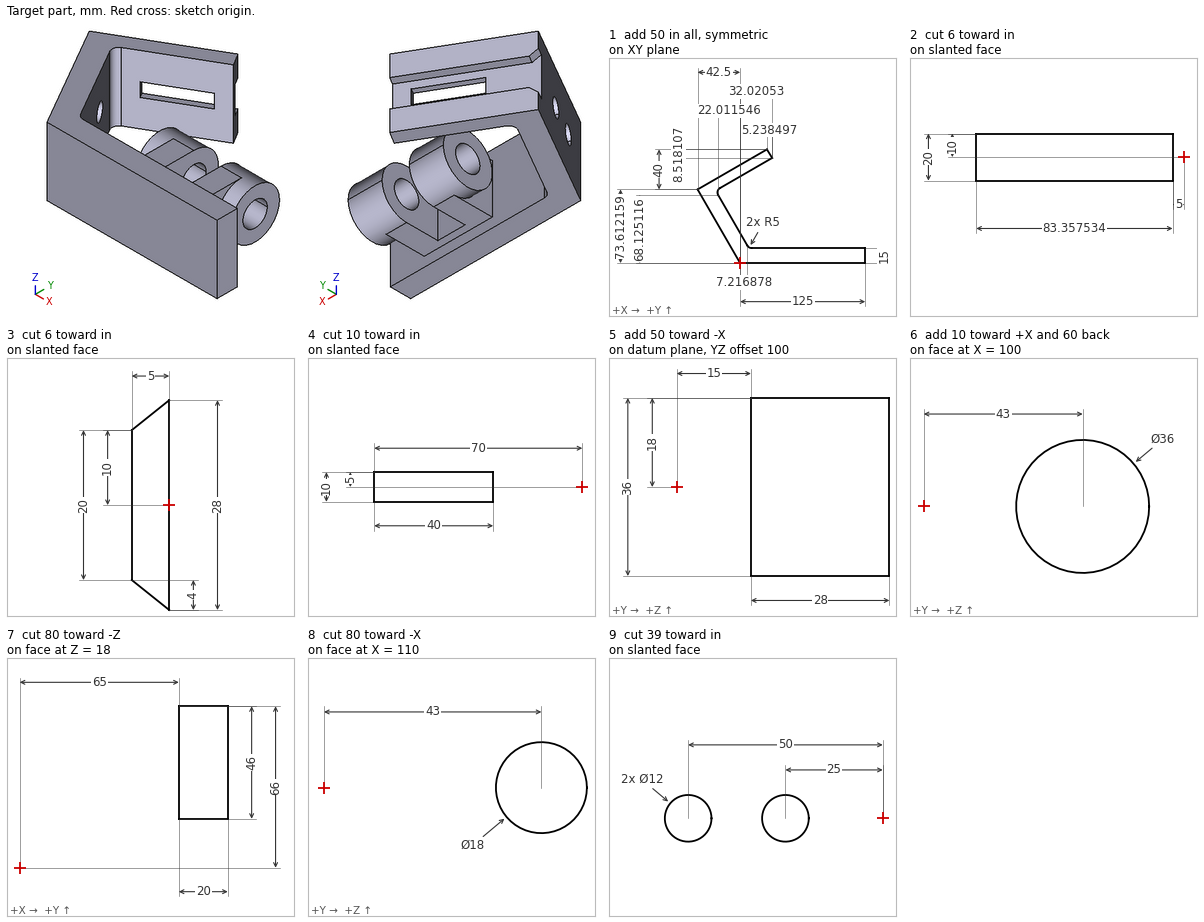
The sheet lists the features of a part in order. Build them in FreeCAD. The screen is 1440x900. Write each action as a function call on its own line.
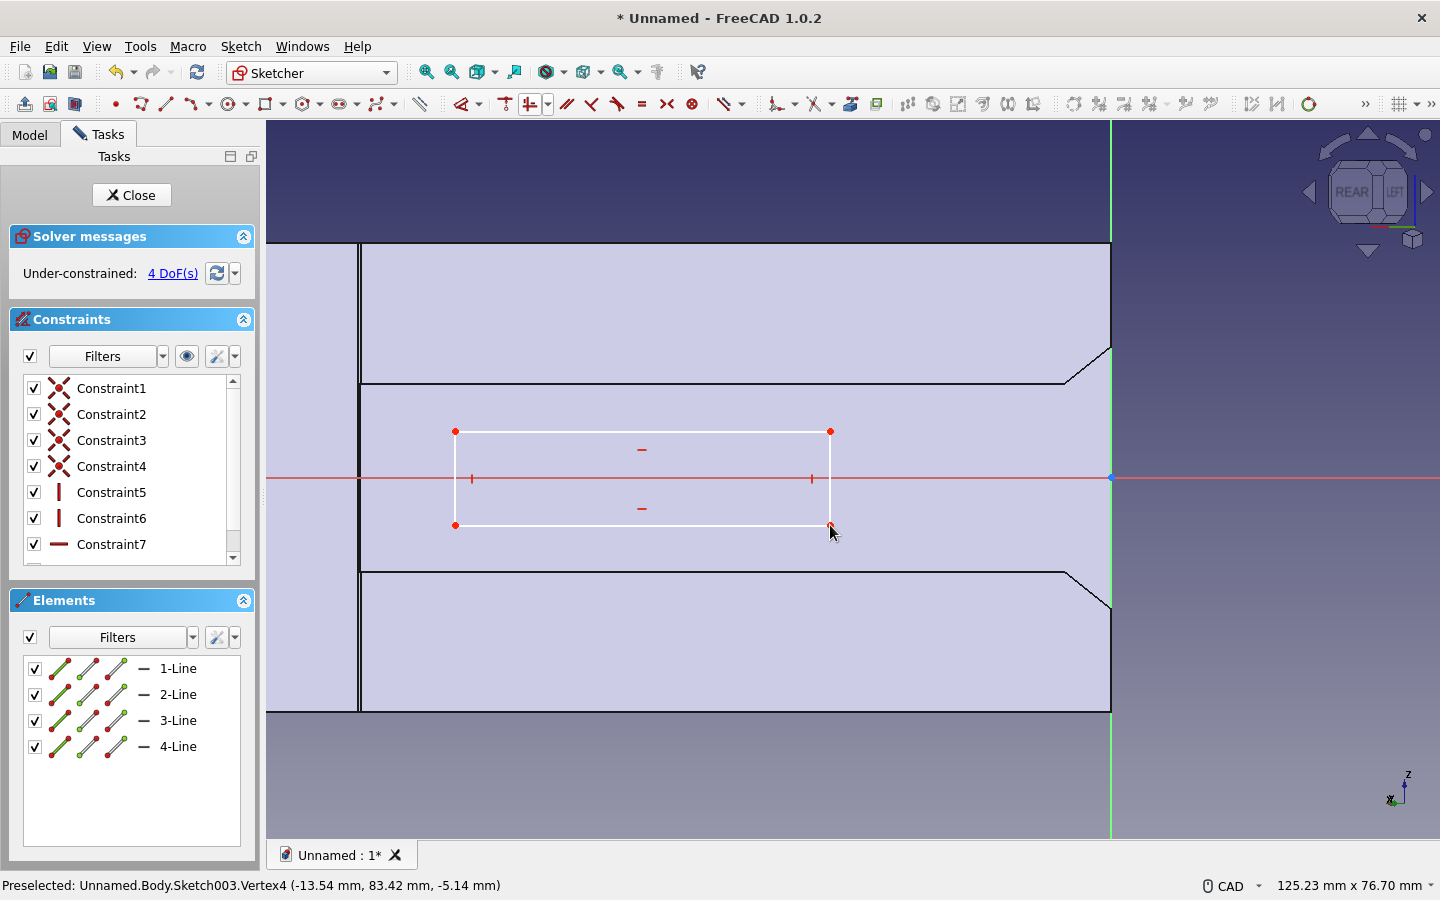
key(d)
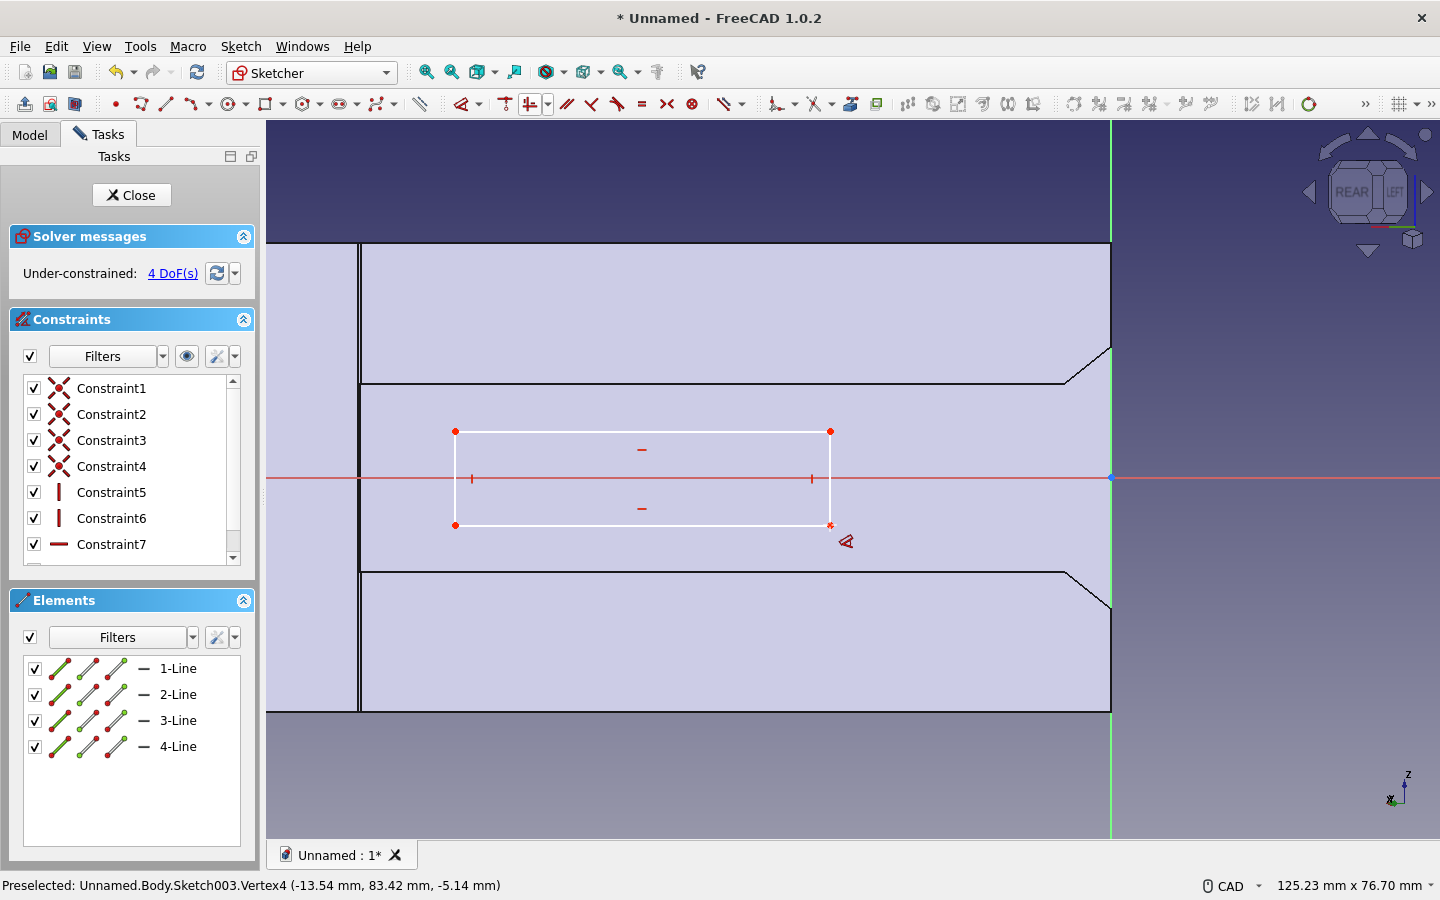
click(455, 460)
click(421, 457)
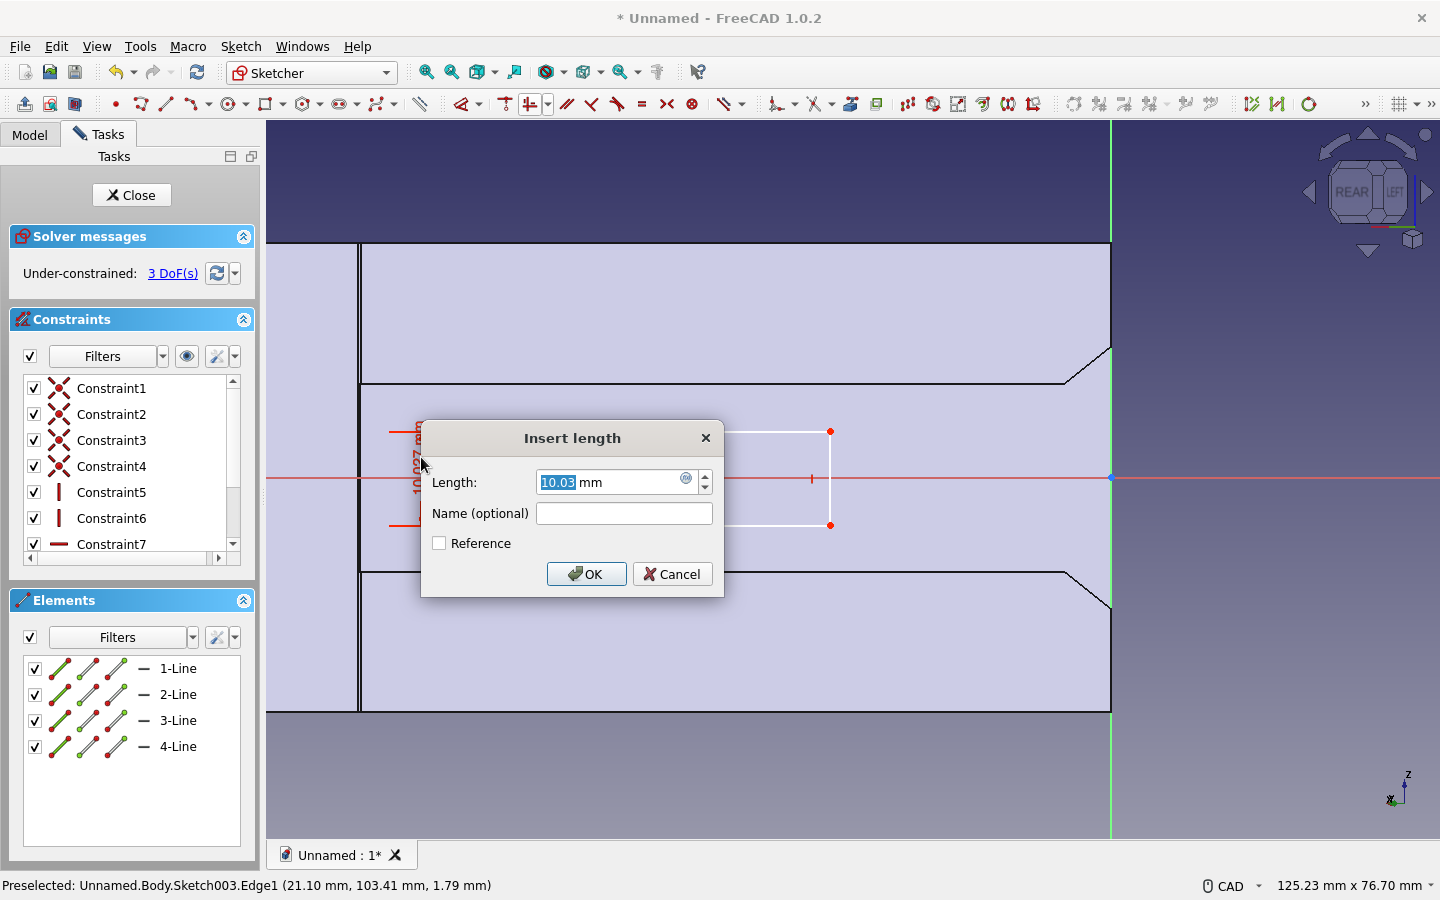
text(10)
key(Return)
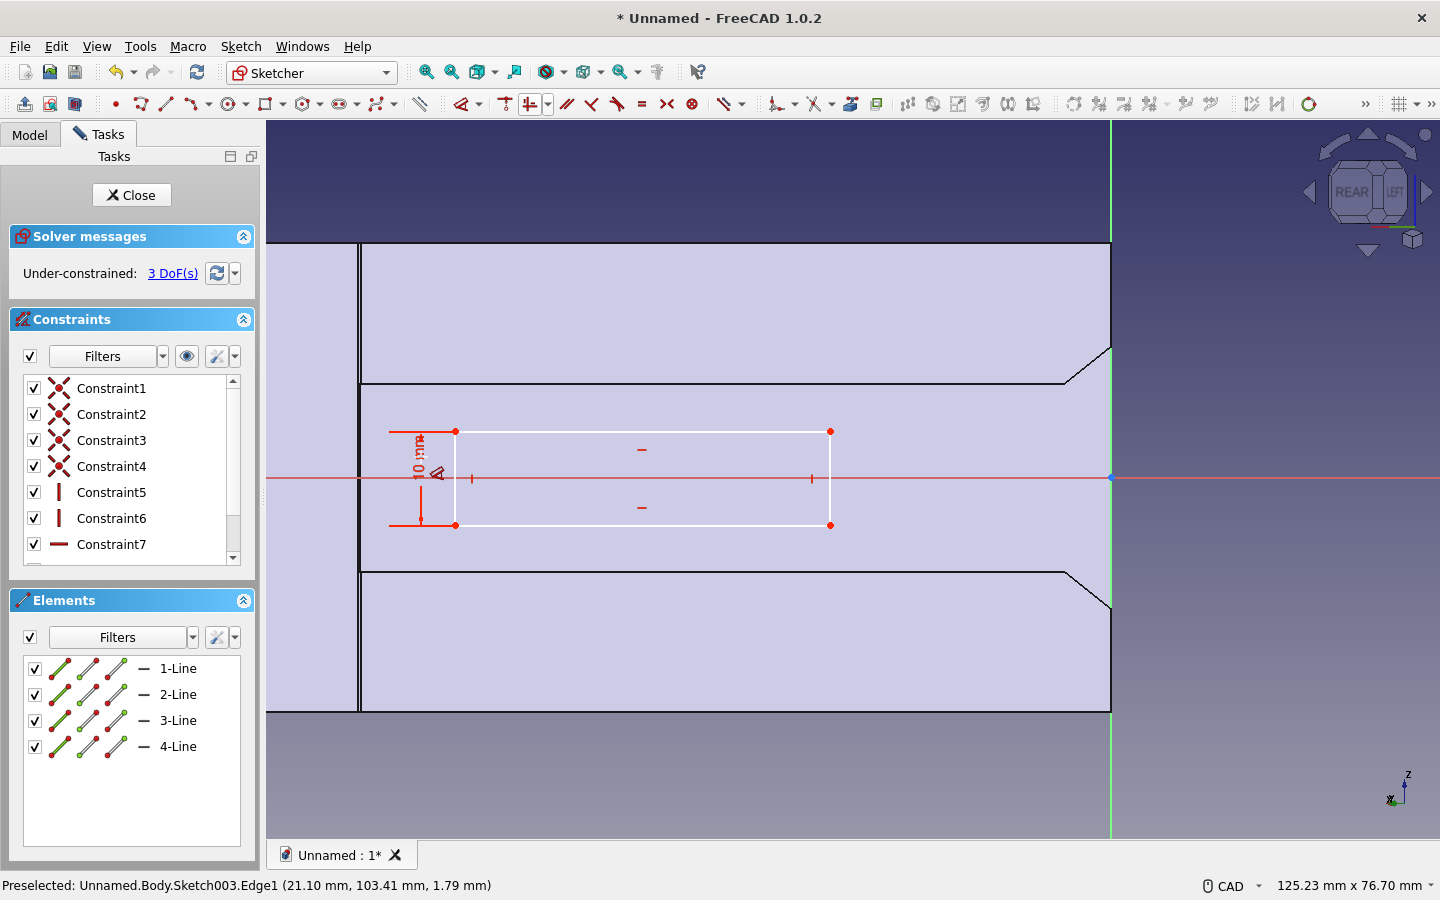
click(567, 526)
click(642, 560)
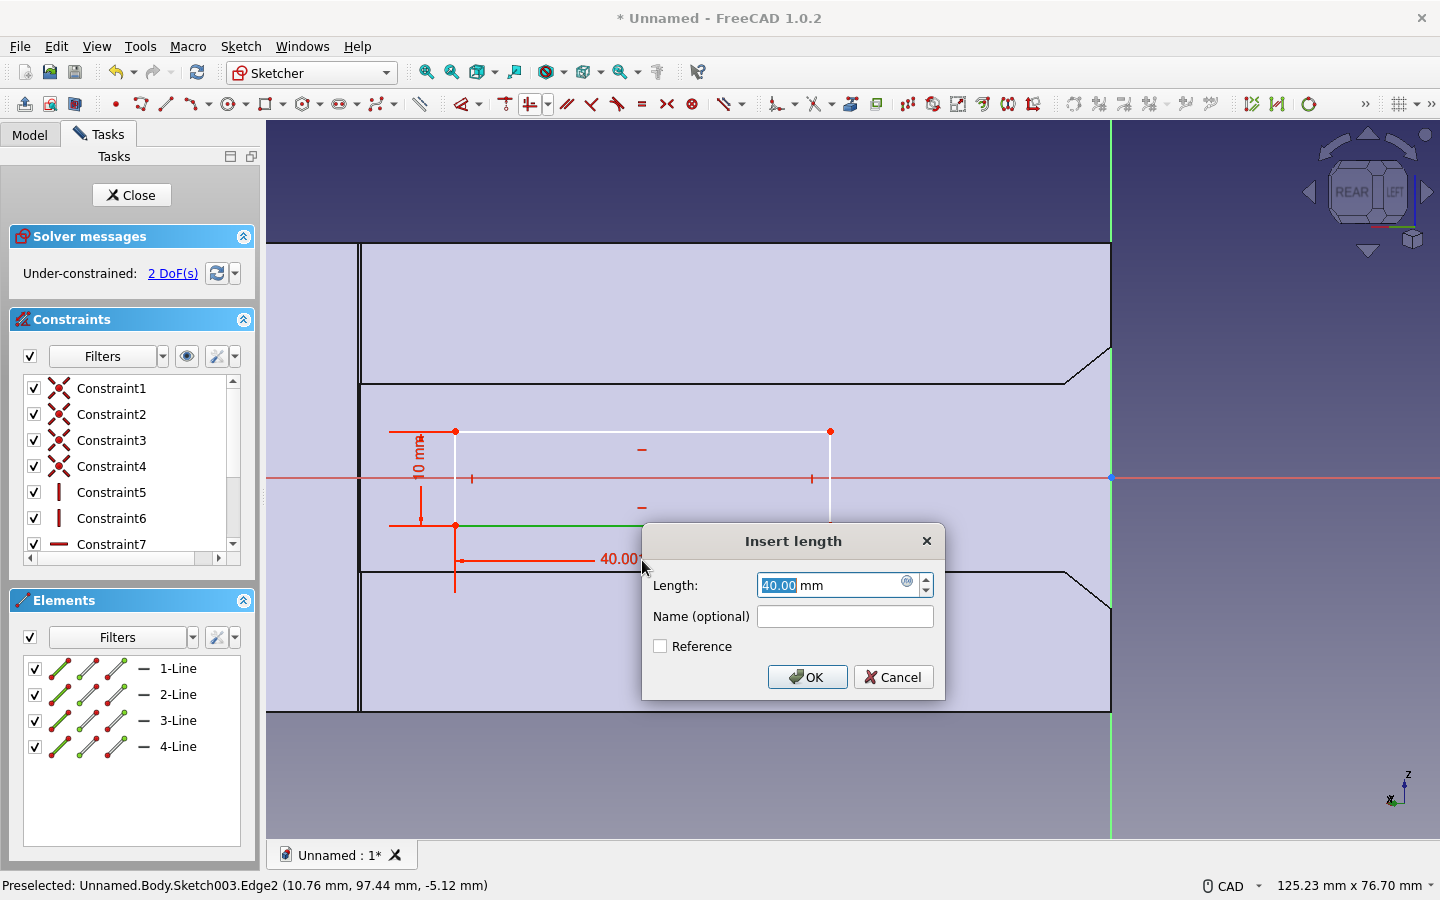
text(40)
key(Return)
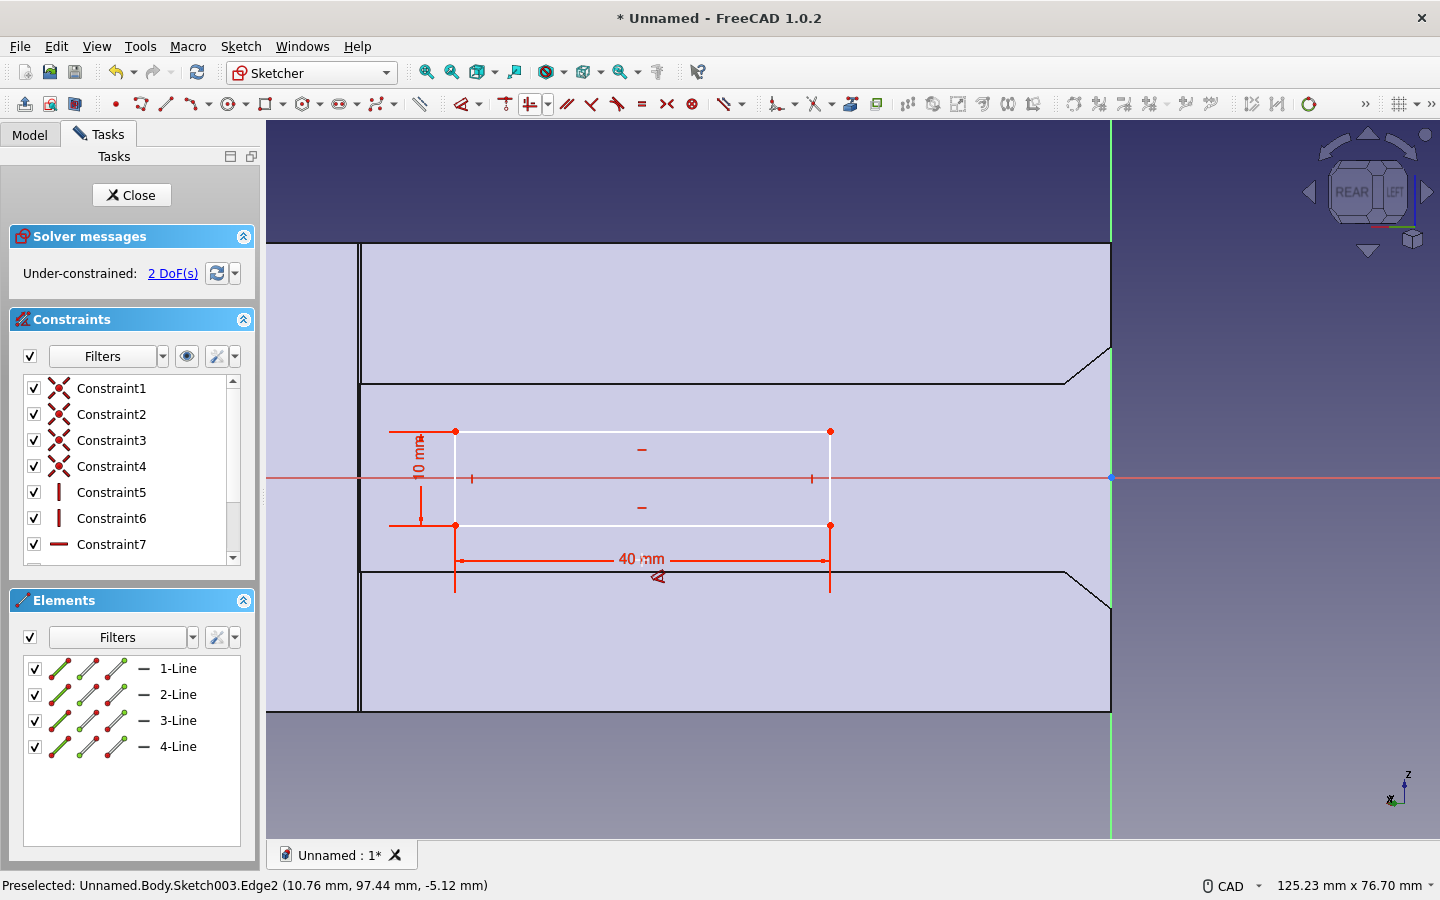
click(455, 432)
click(1145, 455)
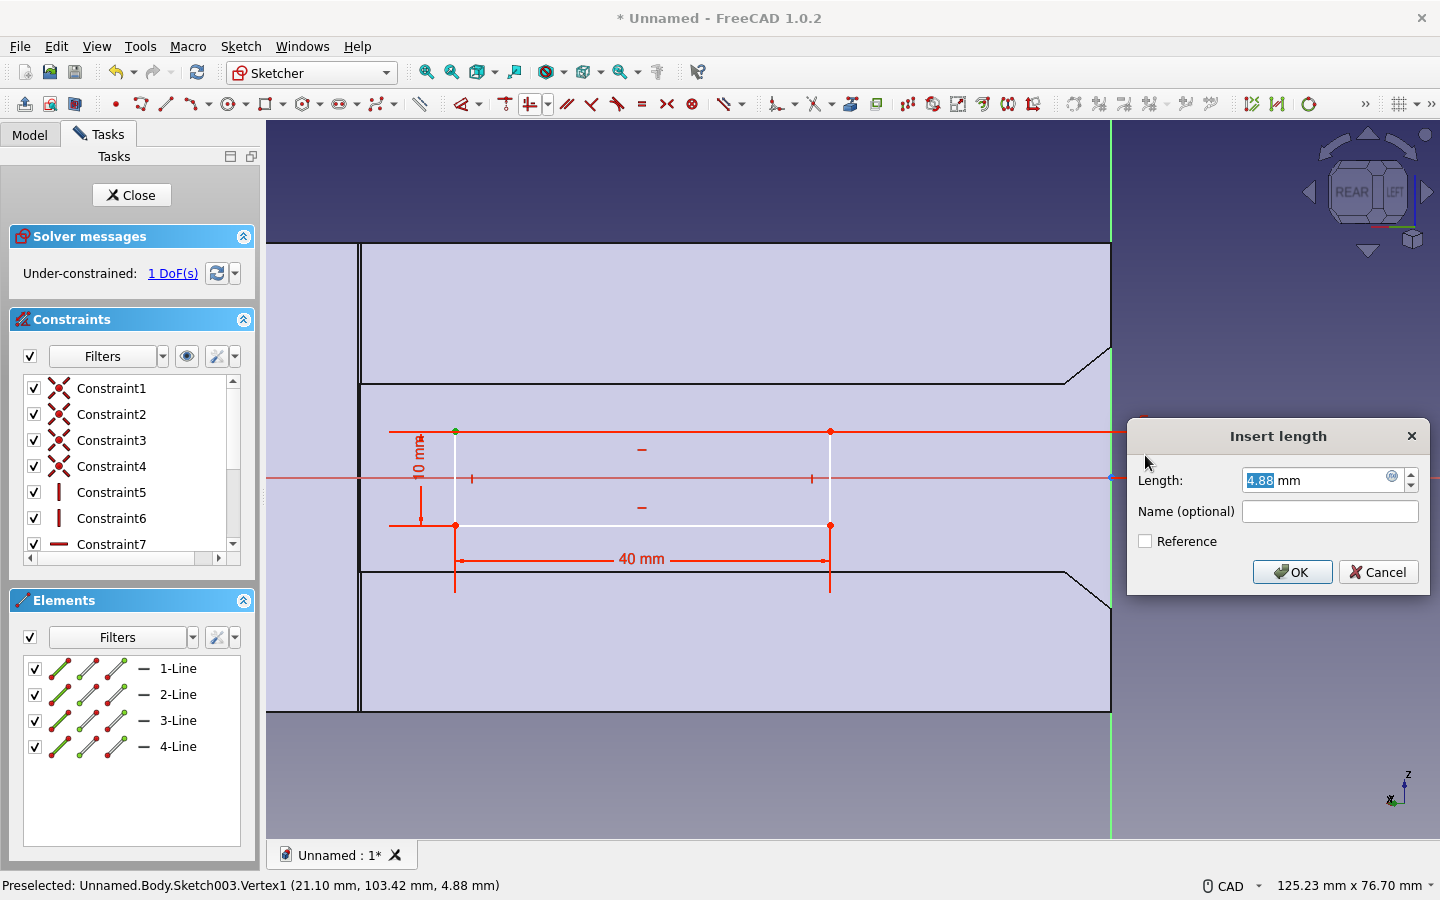
text(5)
key(Return)